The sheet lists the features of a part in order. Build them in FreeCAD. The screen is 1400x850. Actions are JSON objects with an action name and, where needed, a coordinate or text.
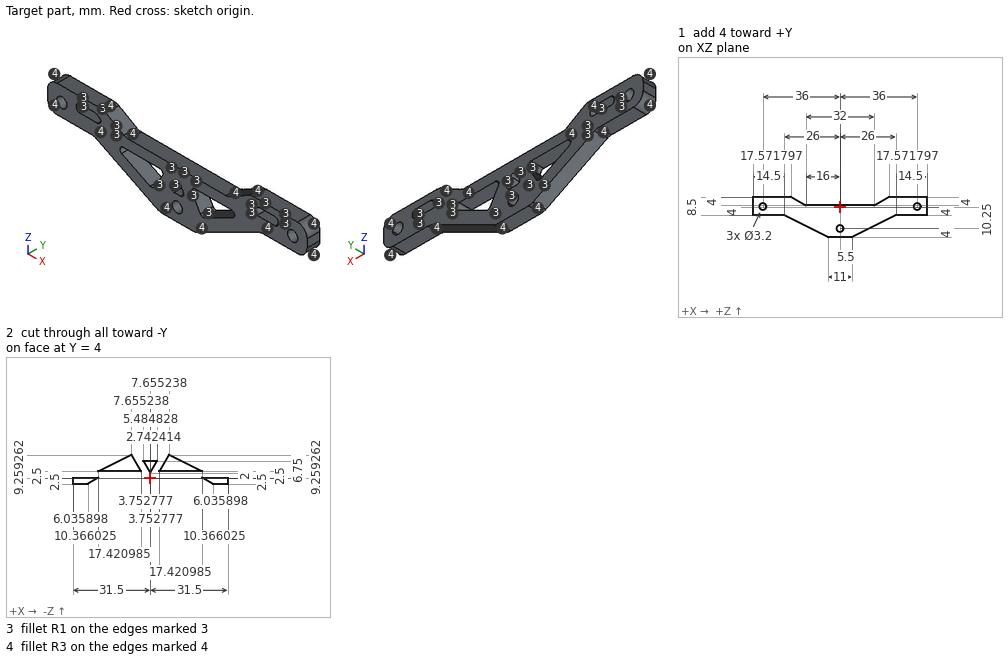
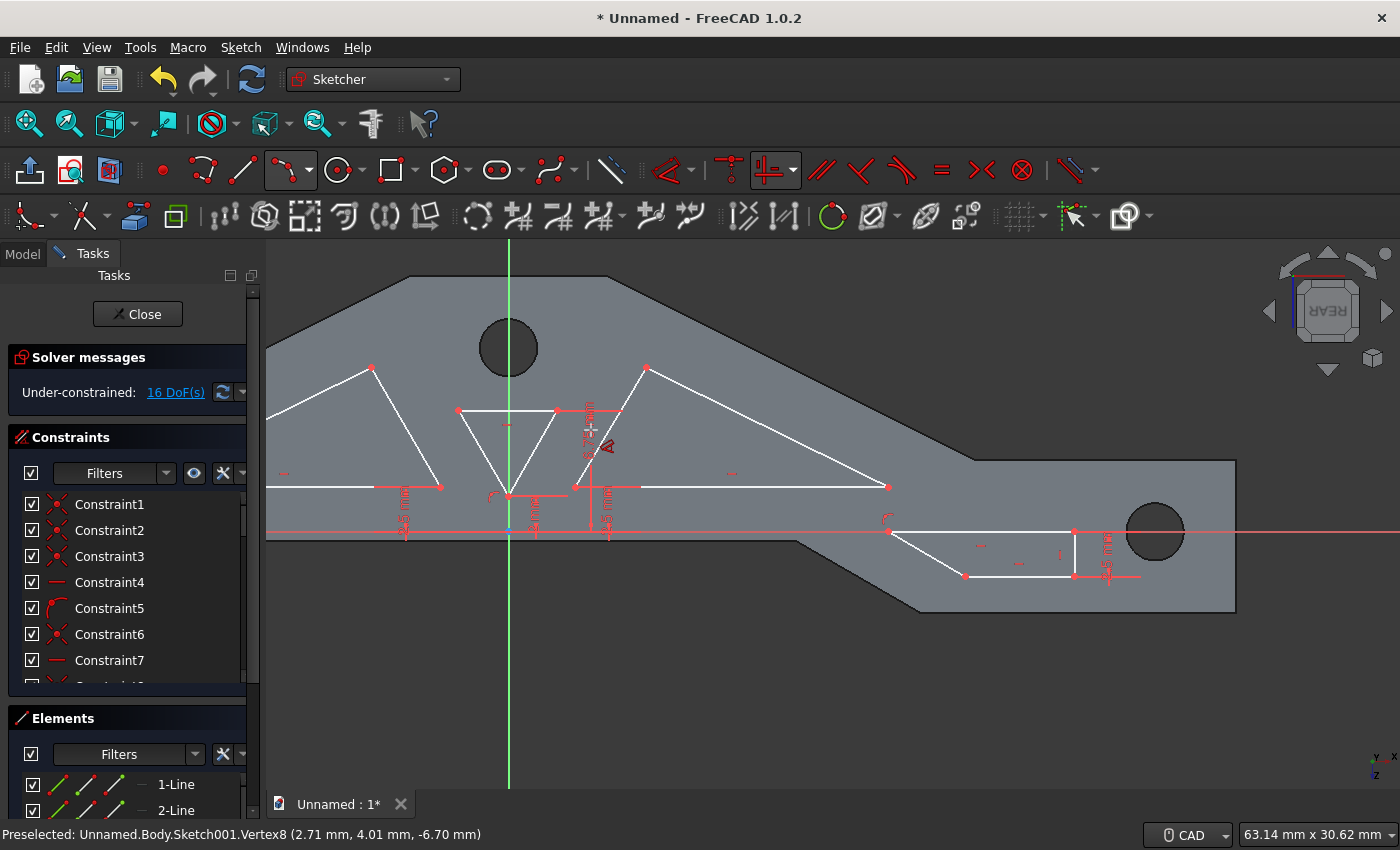
{"action": "scroll", "coordinate": [1076, 566], "scroll_direction": "down", "scroll_amount": 3}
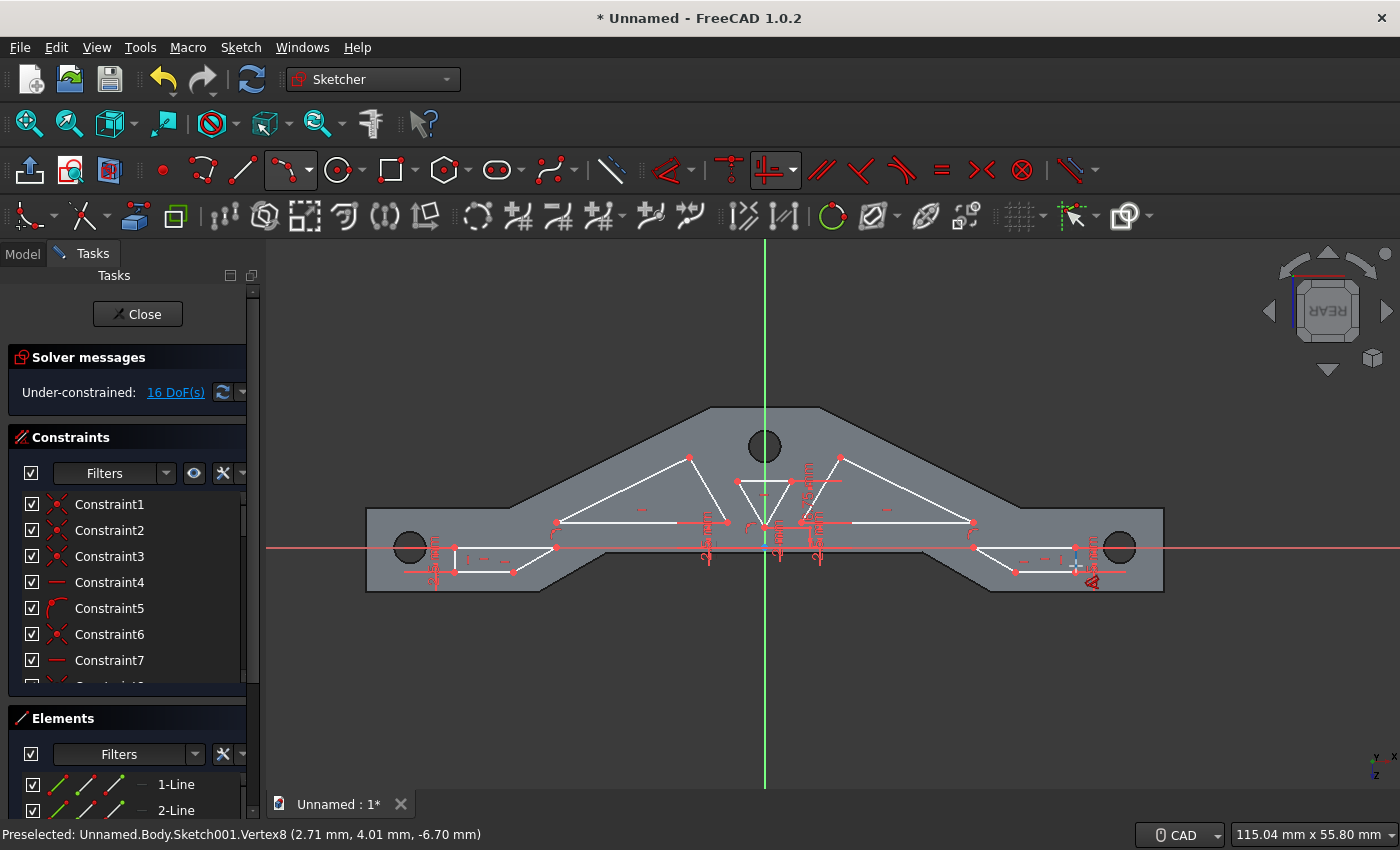
{"action": "left_click", "coordinate": [455, 548]}
{"action": "left_click", "coordinate": [610, 582]}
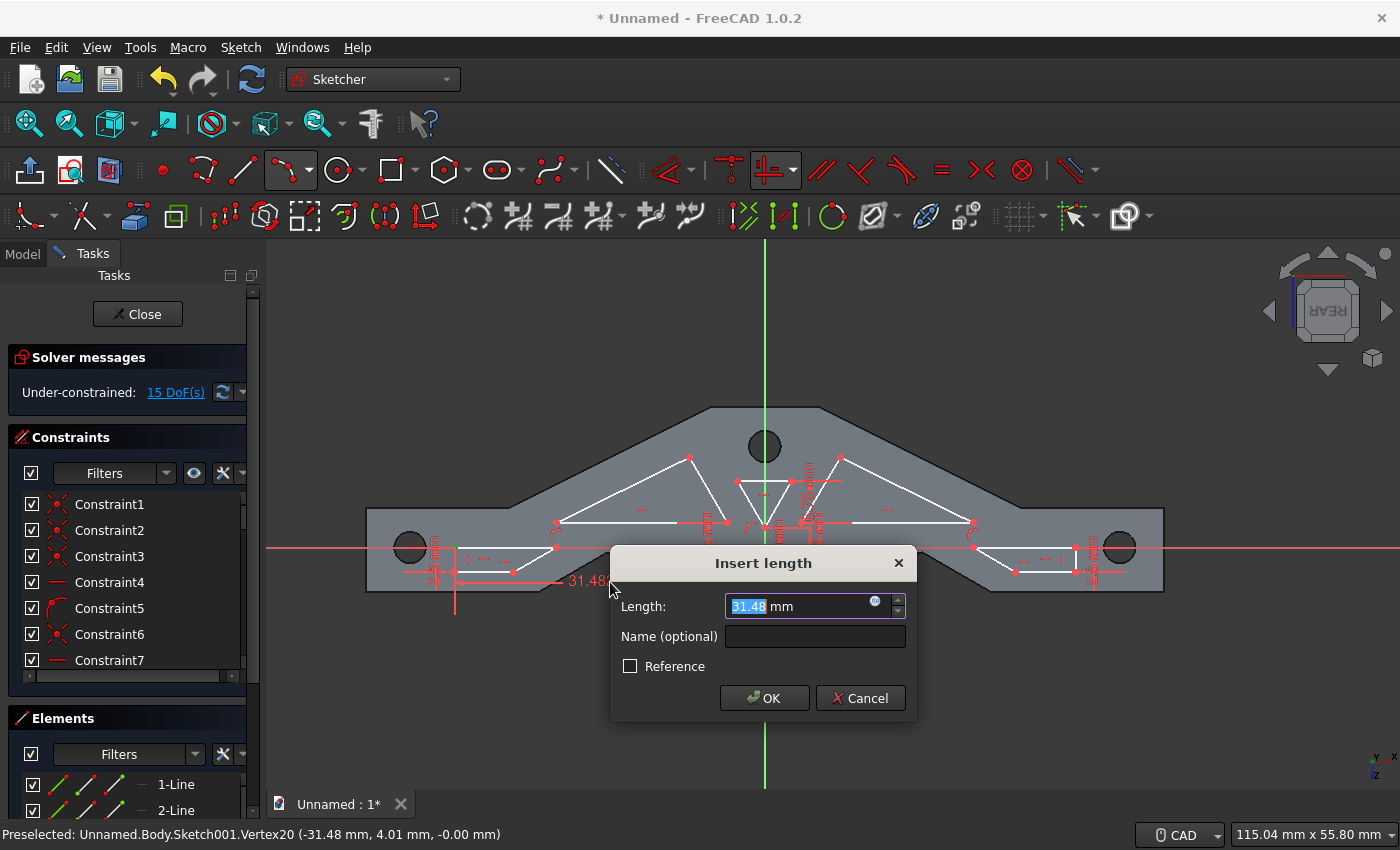
{"action": "type", "text": "31.5"}
{"action": "key", "text": "Return"}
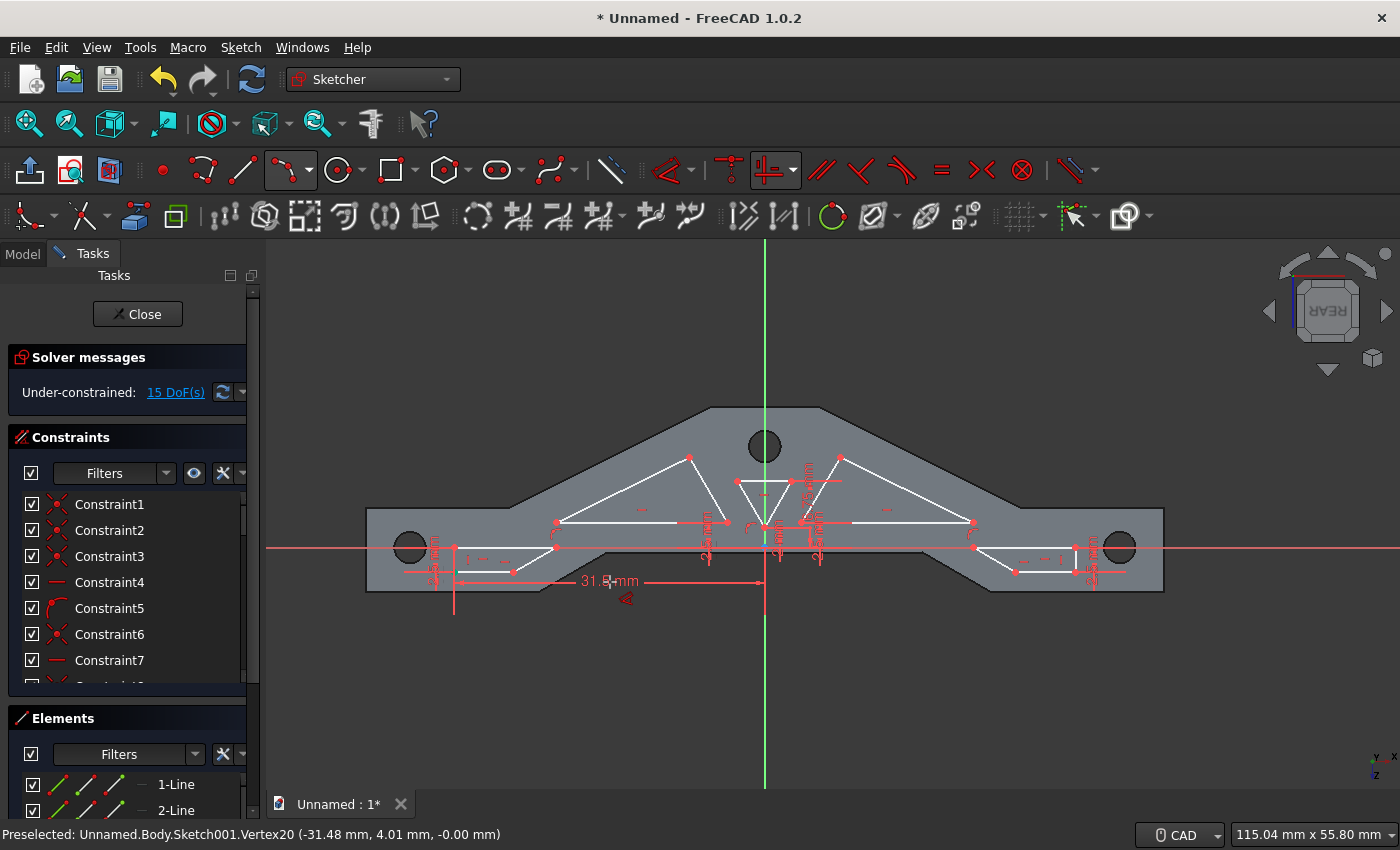
{"action": "left_click", "coordinate": [1076, 572]}
{"action": "left_click", "coordinate": [920, 606]}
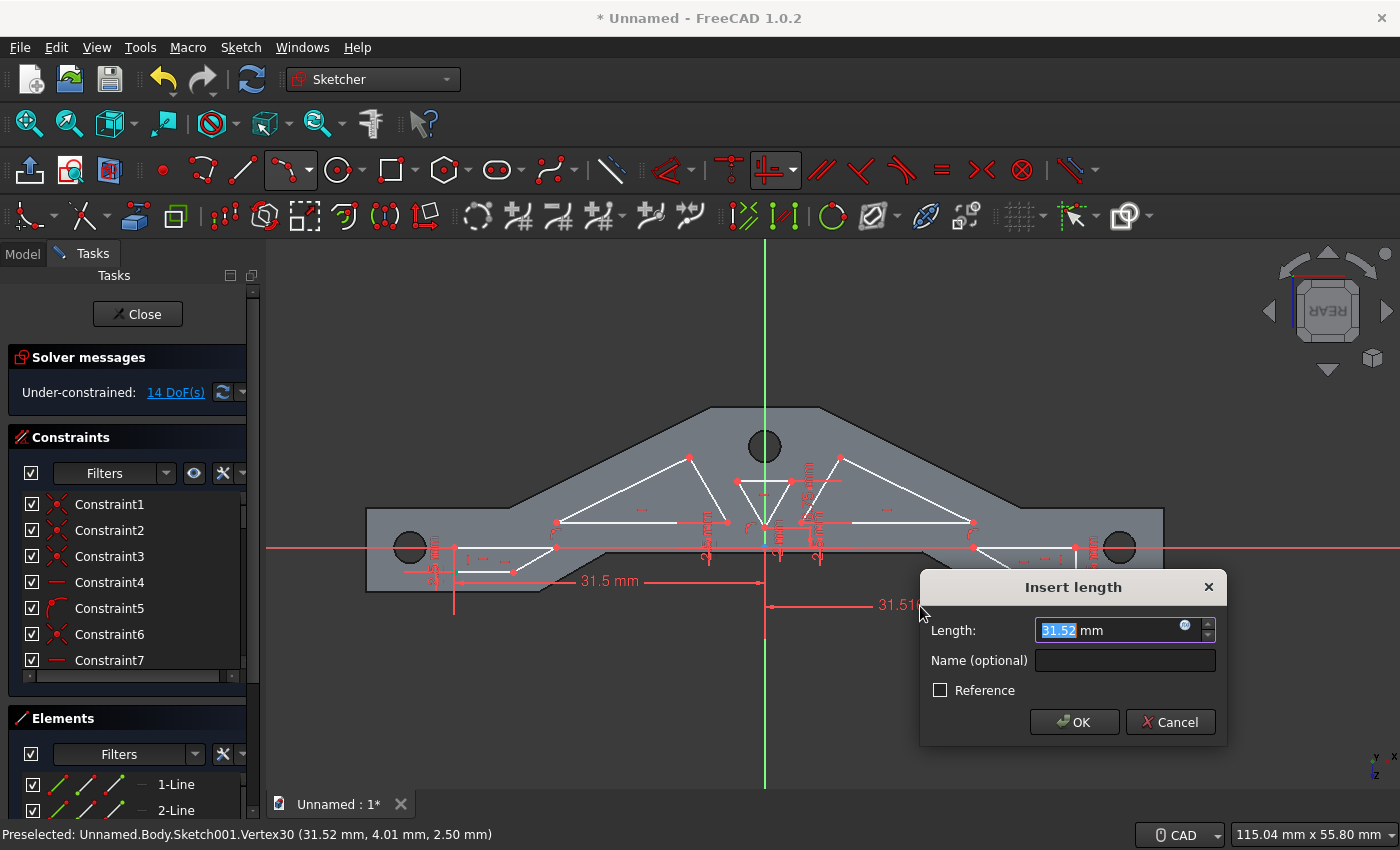
{"action": "type", "text": "31.5"}
{"action": "key", "text": "Return"}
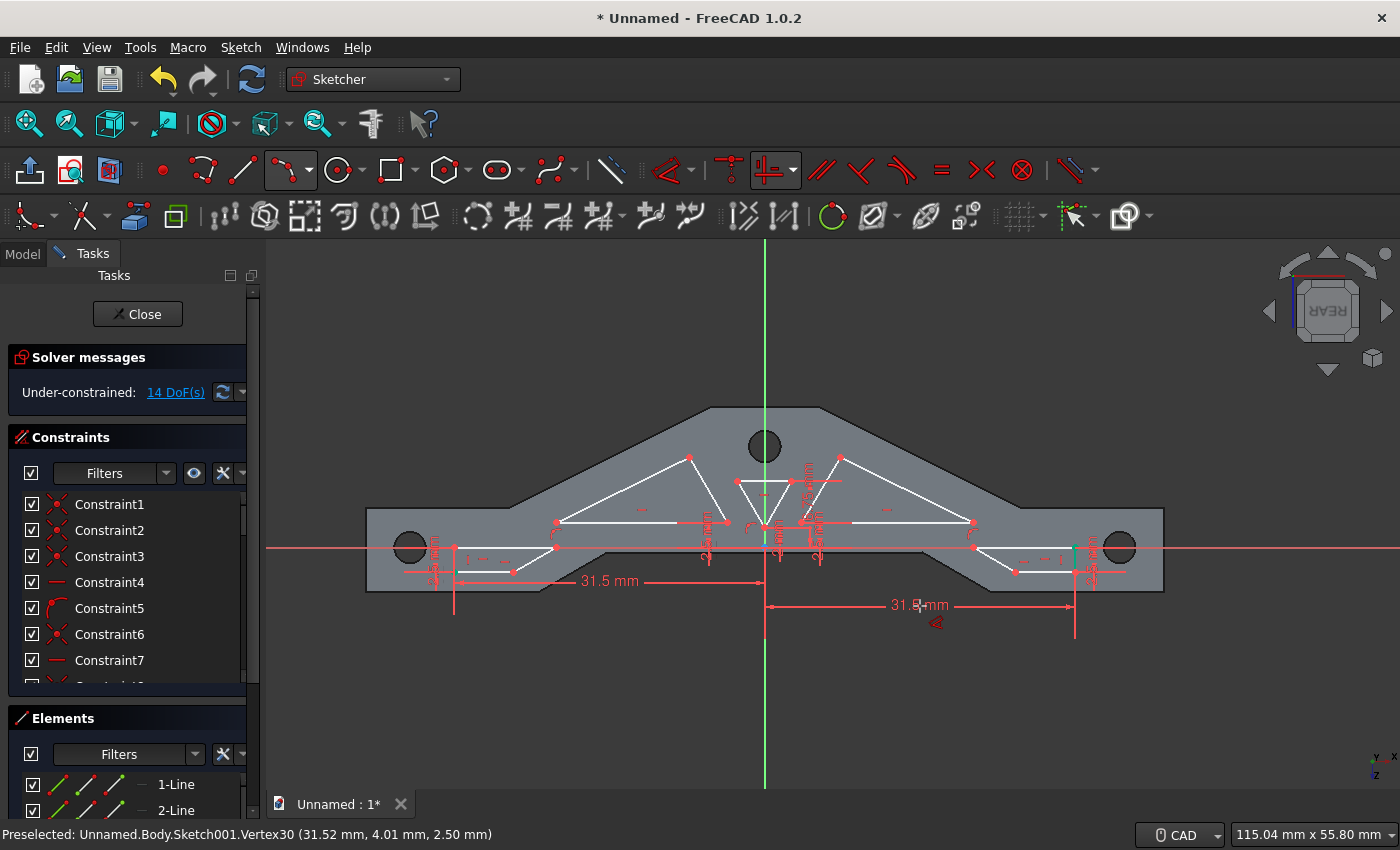
{"action": "scroll", "coordinate": [775, 481], "scroll_direction": "up", "scroll_amount": 2}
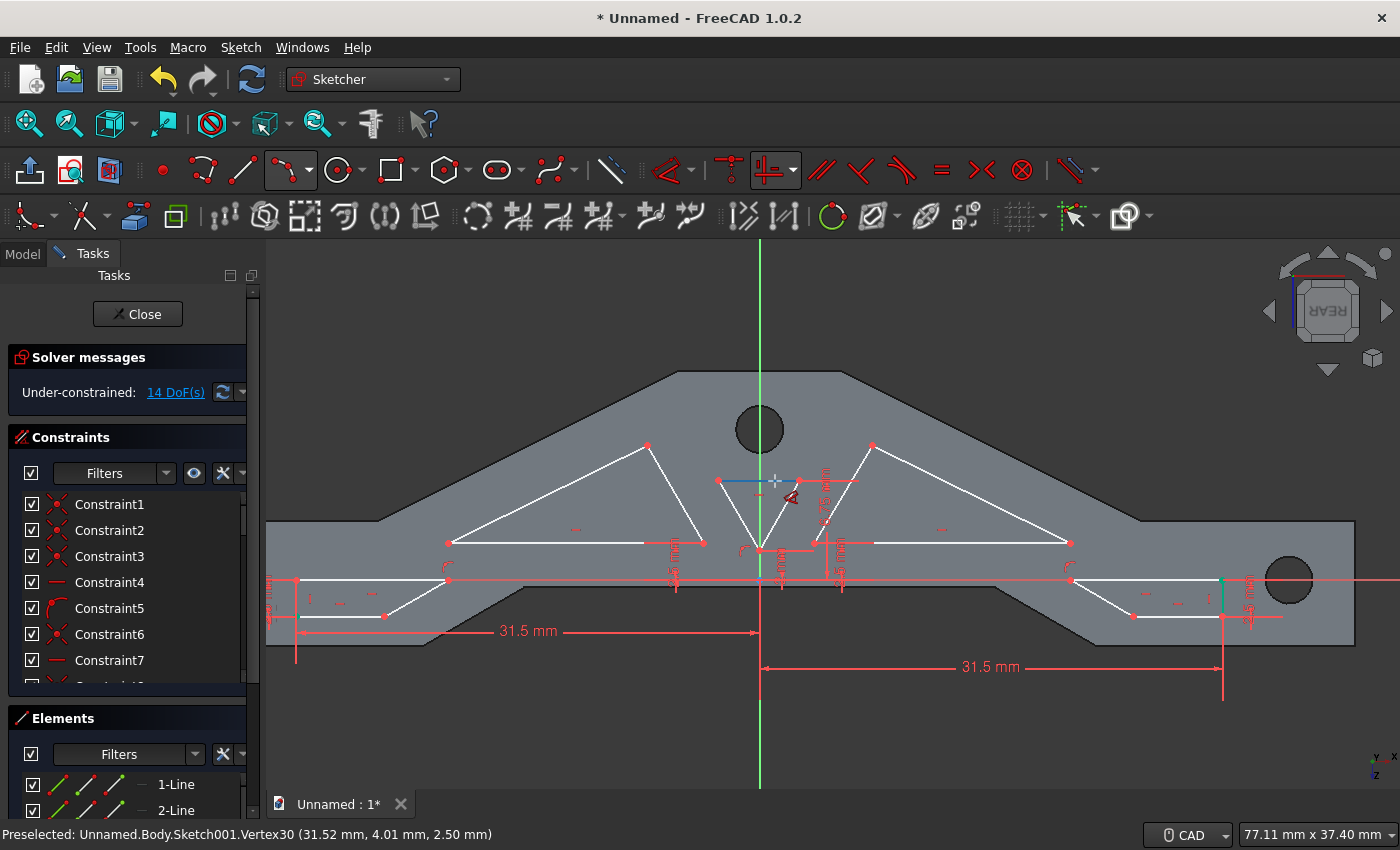
{"action": "left_click", "coordinate": [775, 481]}
{"action": "left_click", "coordinate": [741, 447]}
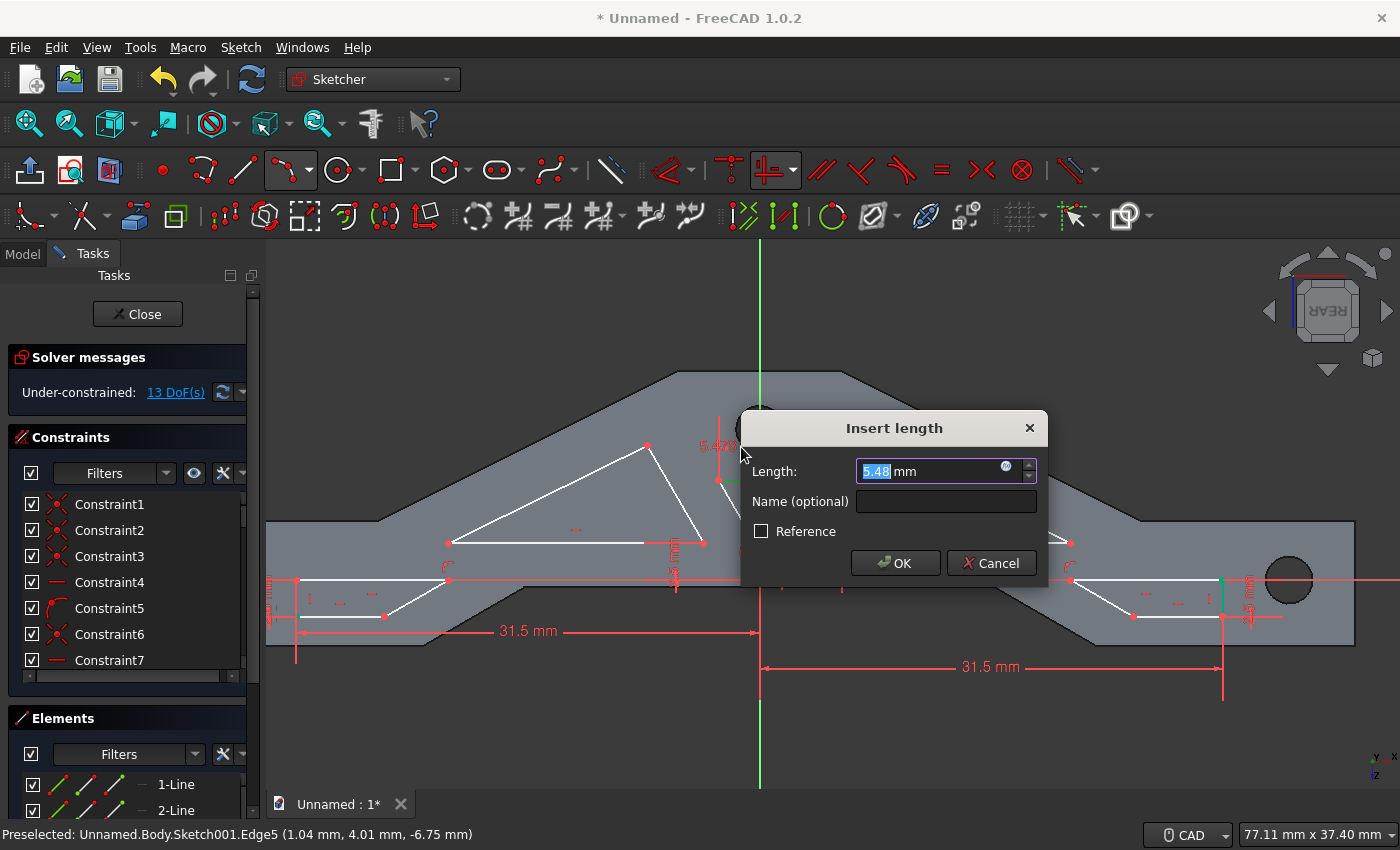
{"action": "type", "text": "5.484828"}
{"action": "key", "text": "Return"}